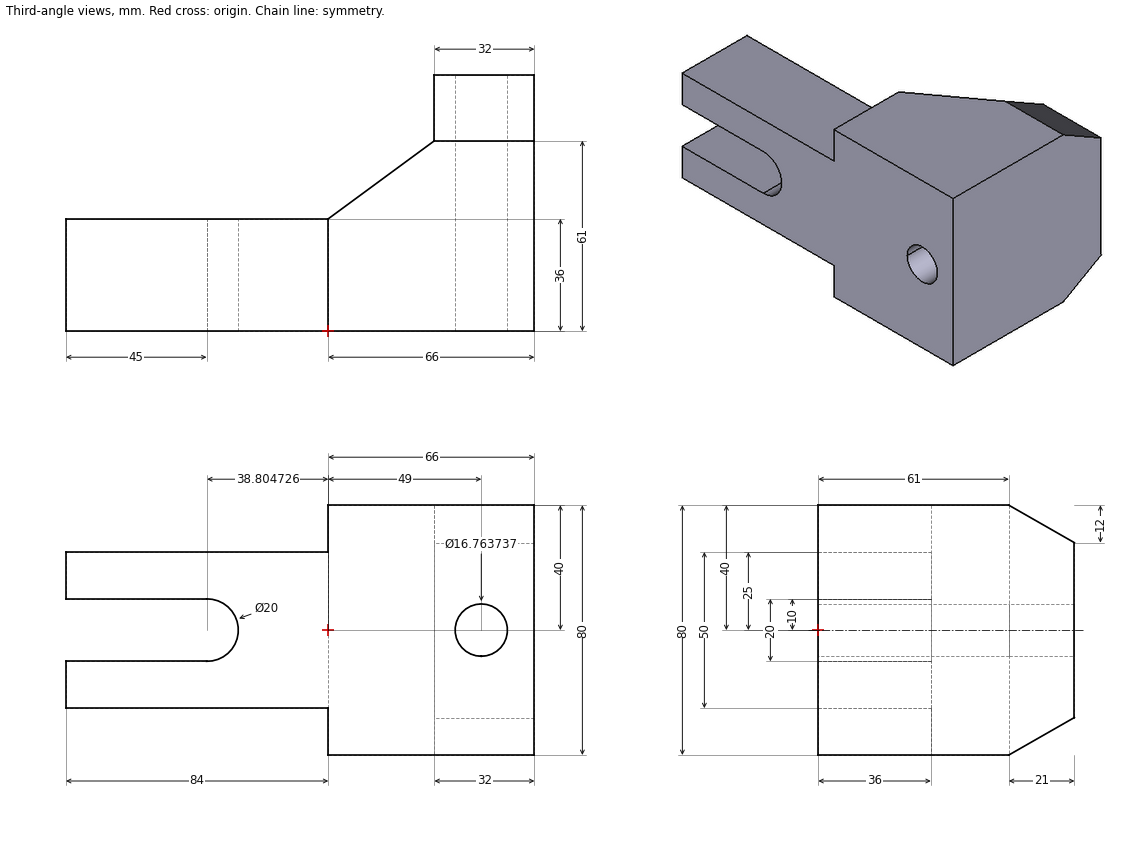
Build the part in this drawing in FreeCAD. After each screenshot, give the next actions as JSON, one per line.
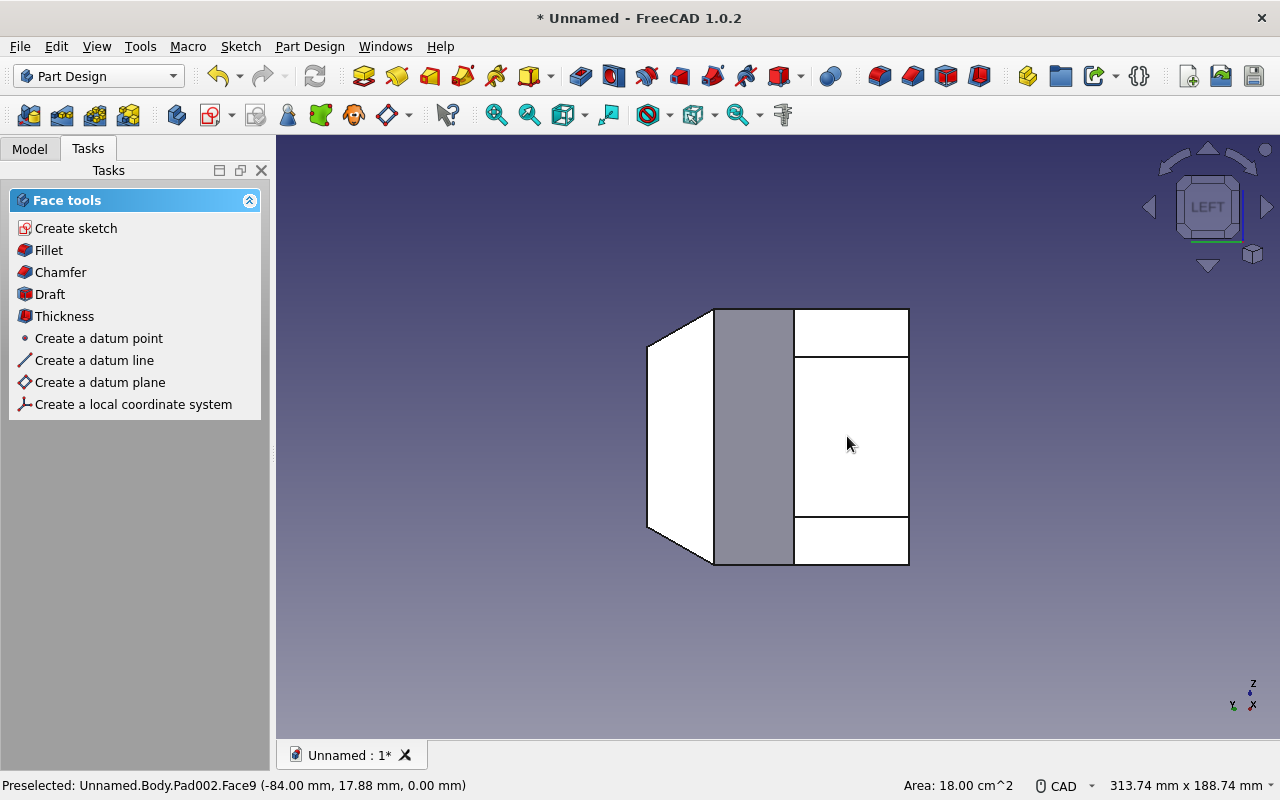
{"action": "left_click", "coordinate": [210, 116]}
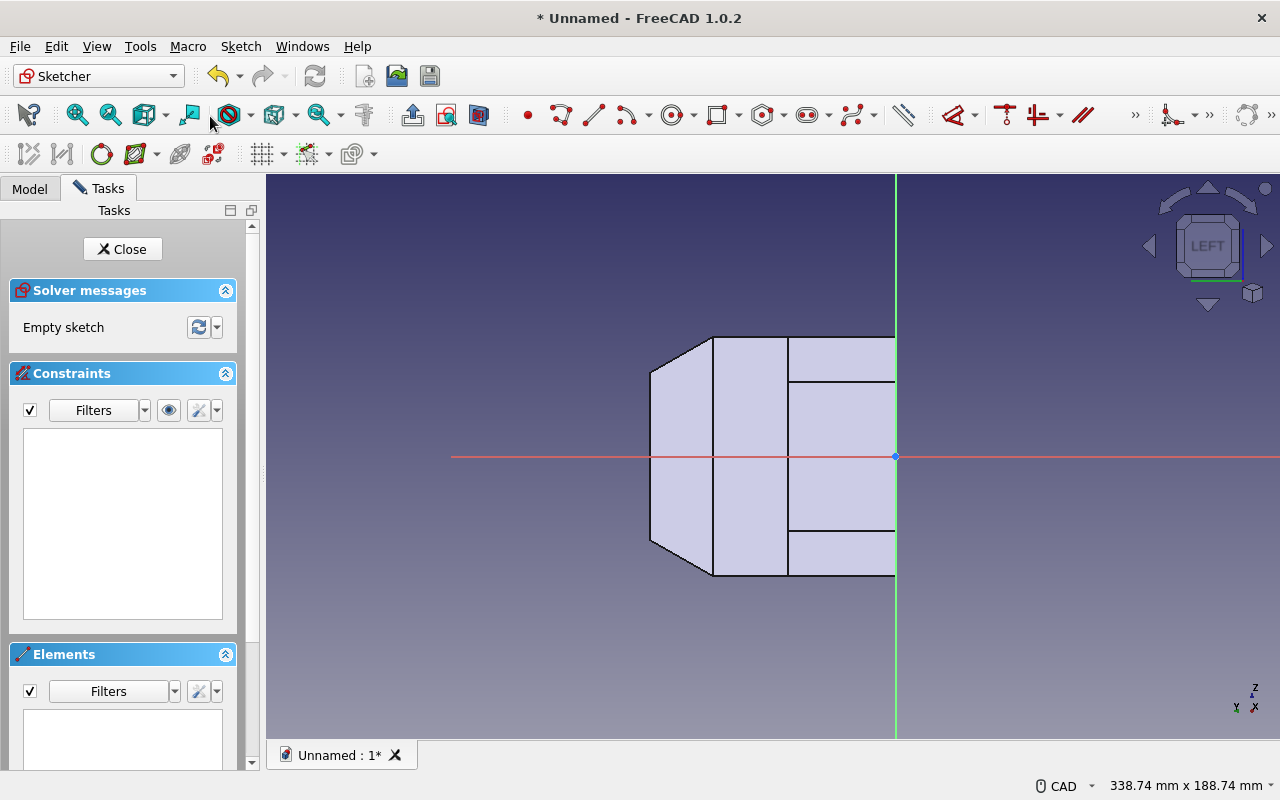
{"action": "scroll", "coordinate": [877, 456], "scroll_direction": "up", "scroll_amount": 8}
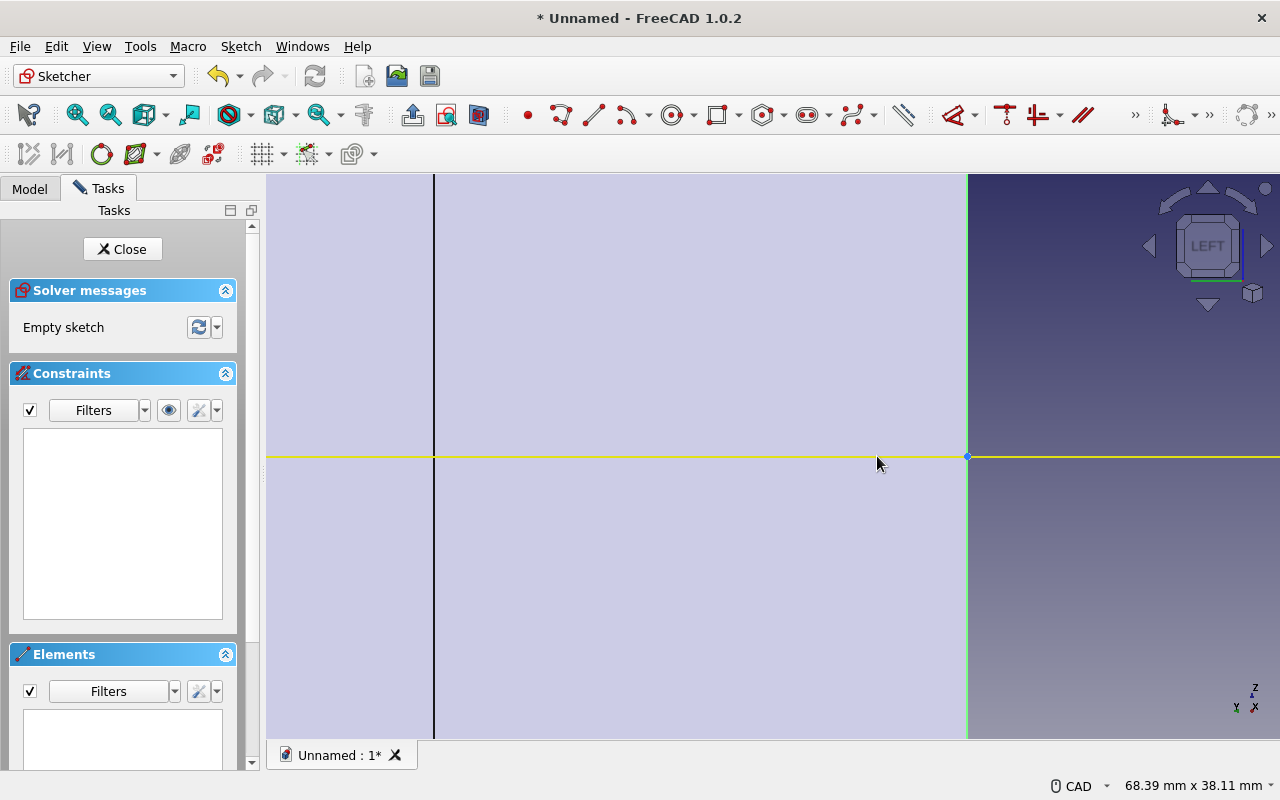
{"action": "key", "text": "g r"}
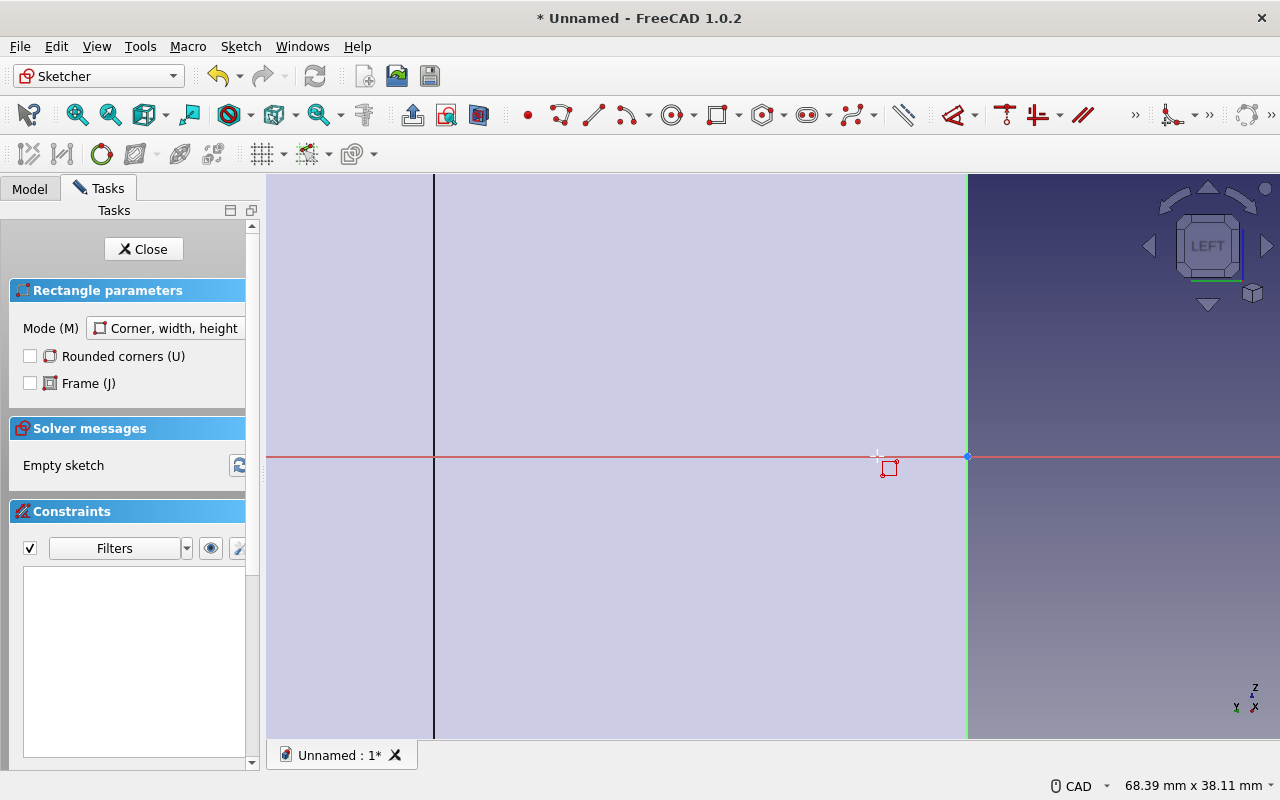
{"action": "left_click", "coordinate": [434, 308]}
{"action": "left_click", "coordinate": [967, 605]}
{"action": "key", "text": "Escape"}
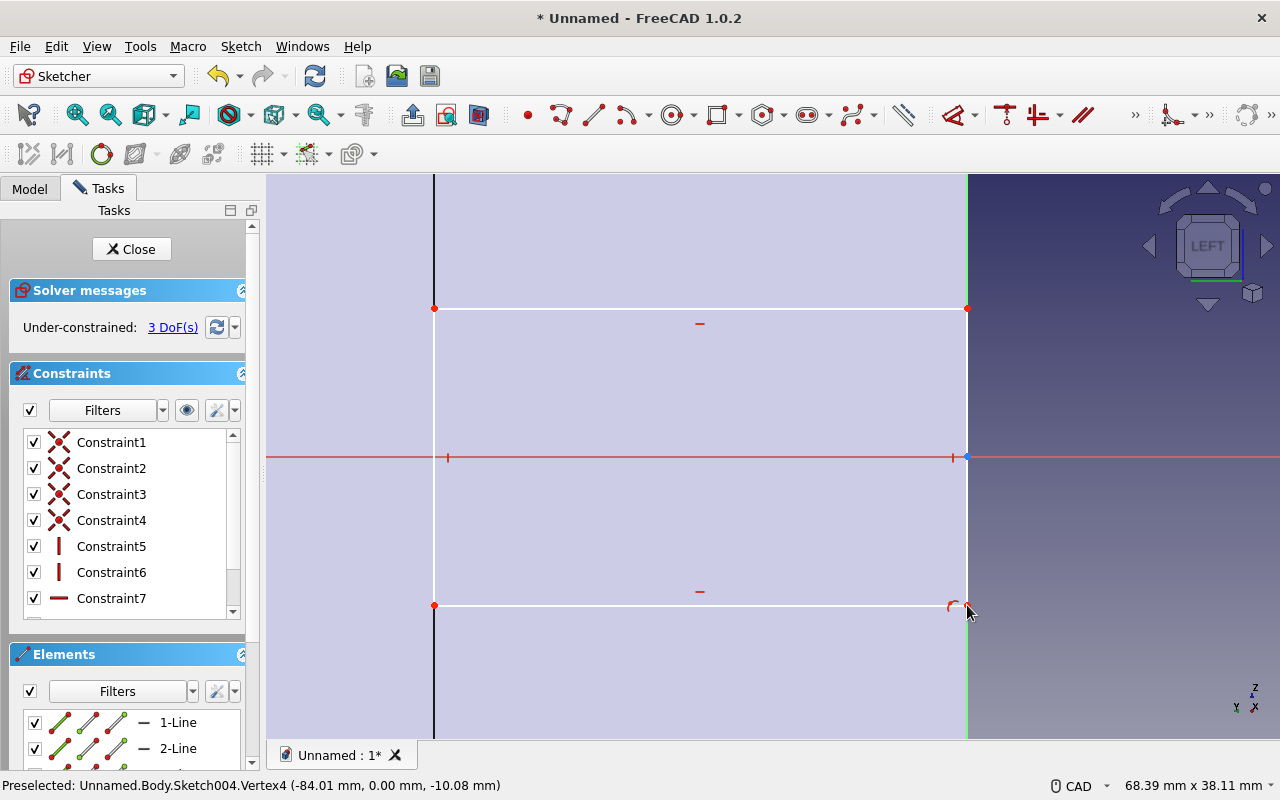
{"action": "left_click", "coordinate": [952, 116]}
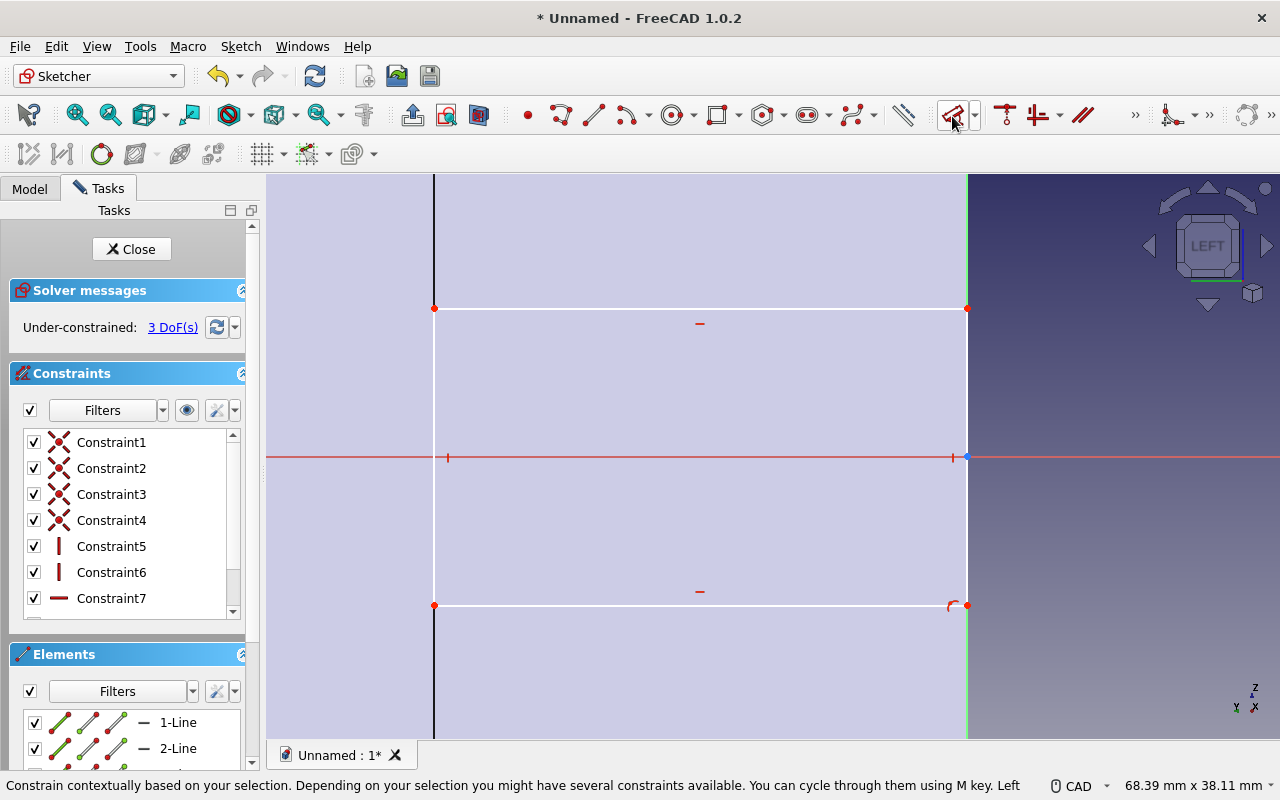
{"action": "left_click", "coordinate": [434, 398]}
{"action": "left_click", "coordinate": [400, 389]}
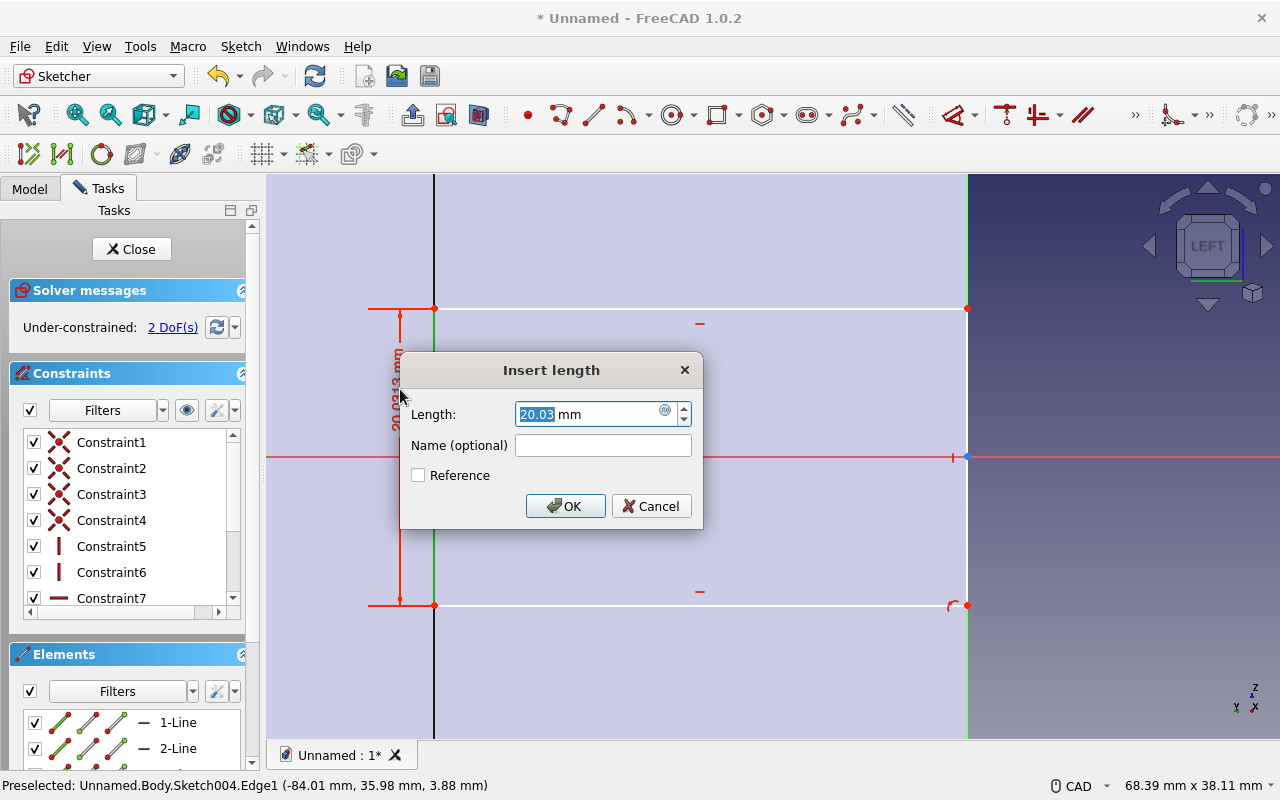
{"action": "type", "text": "20"}
{"action": "key", "text": "Return"}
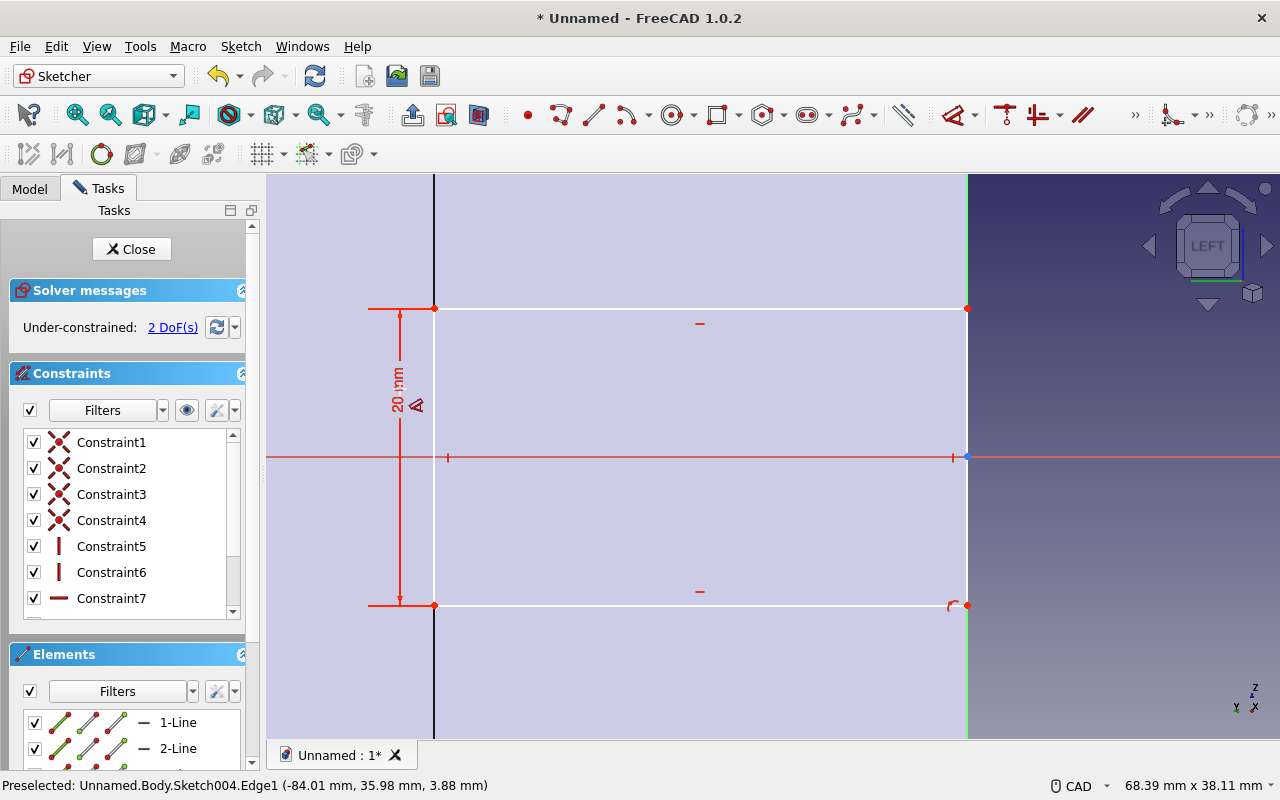
{"action": "left_click", "coordinate": [594, 606]}
{"action": "left_click", "coordinate": [701, 640]}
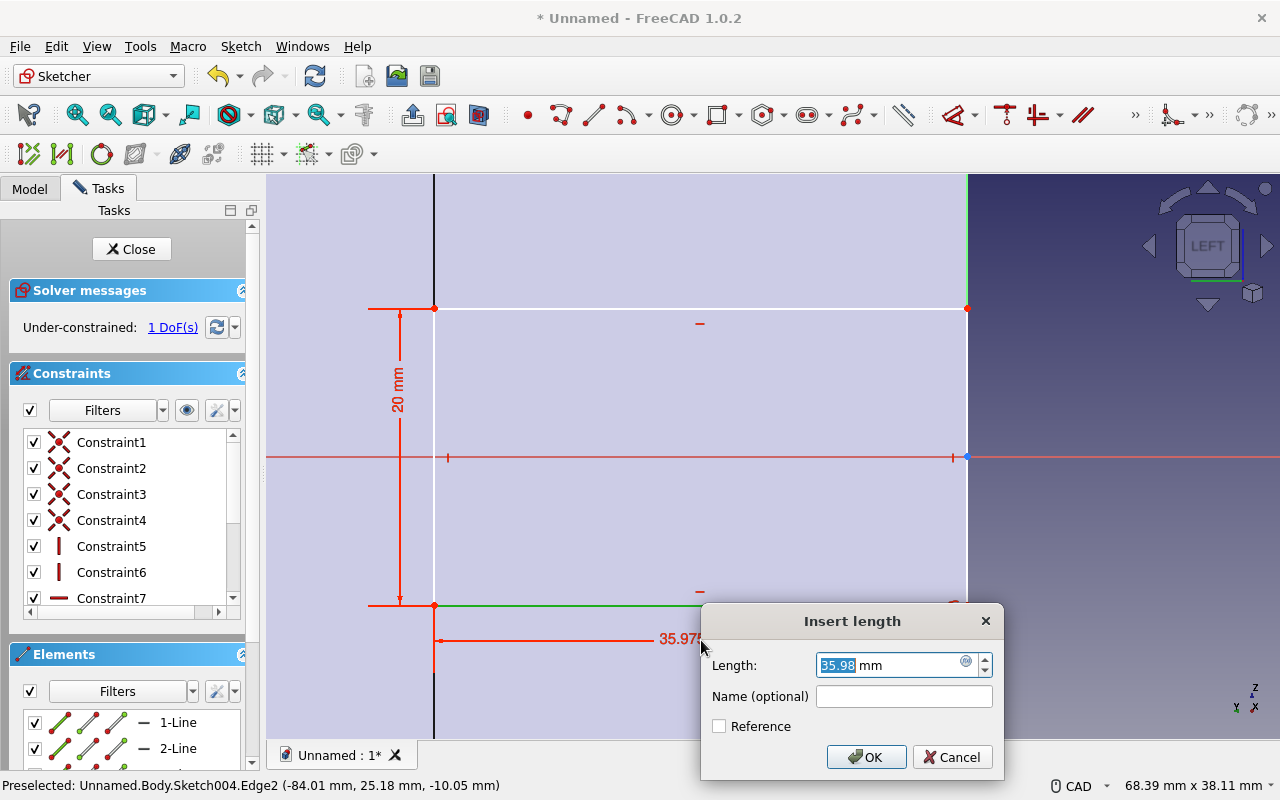
{"action": "type", "text": "36"}
{"action": "key", "text": "Return"}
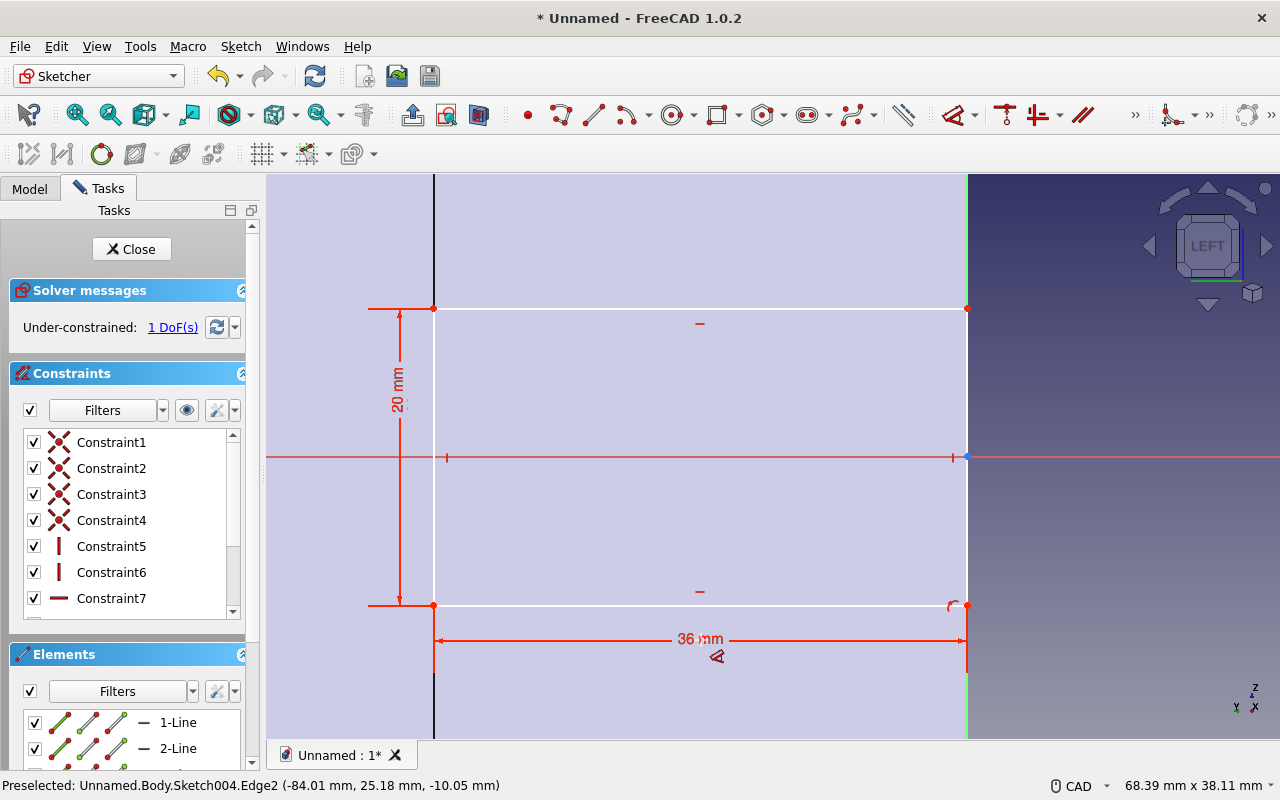
{"action": "left_click", "coordinate": [434, 309]}
{"action": "left_click", "coordinate": [1001, 383]}